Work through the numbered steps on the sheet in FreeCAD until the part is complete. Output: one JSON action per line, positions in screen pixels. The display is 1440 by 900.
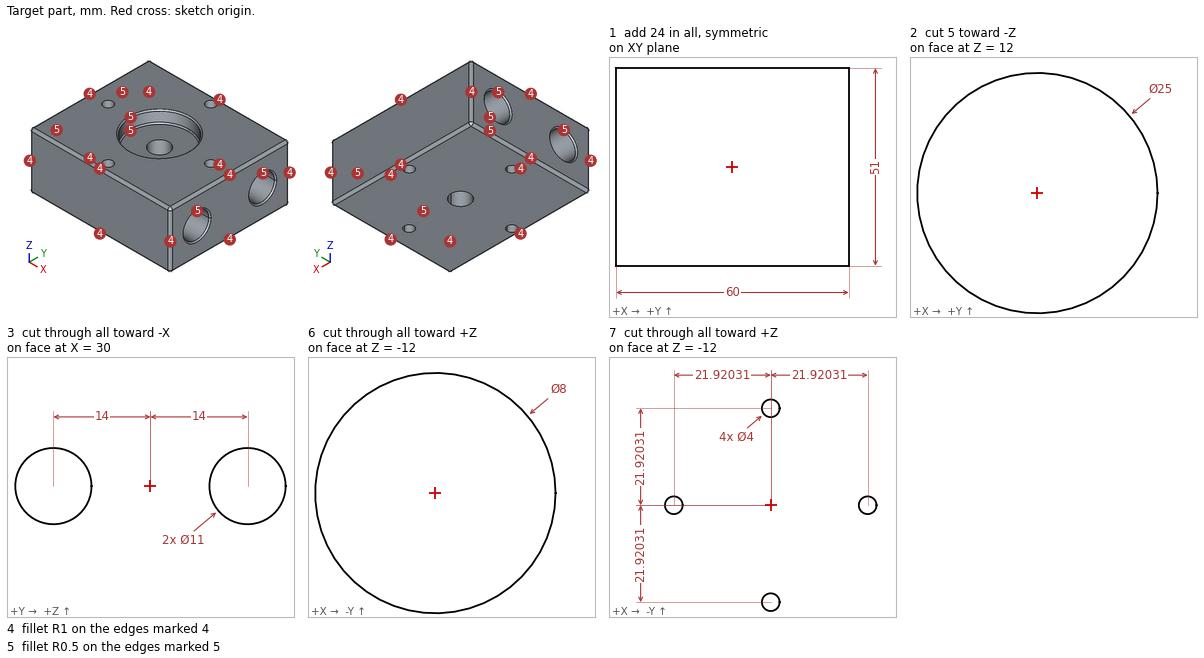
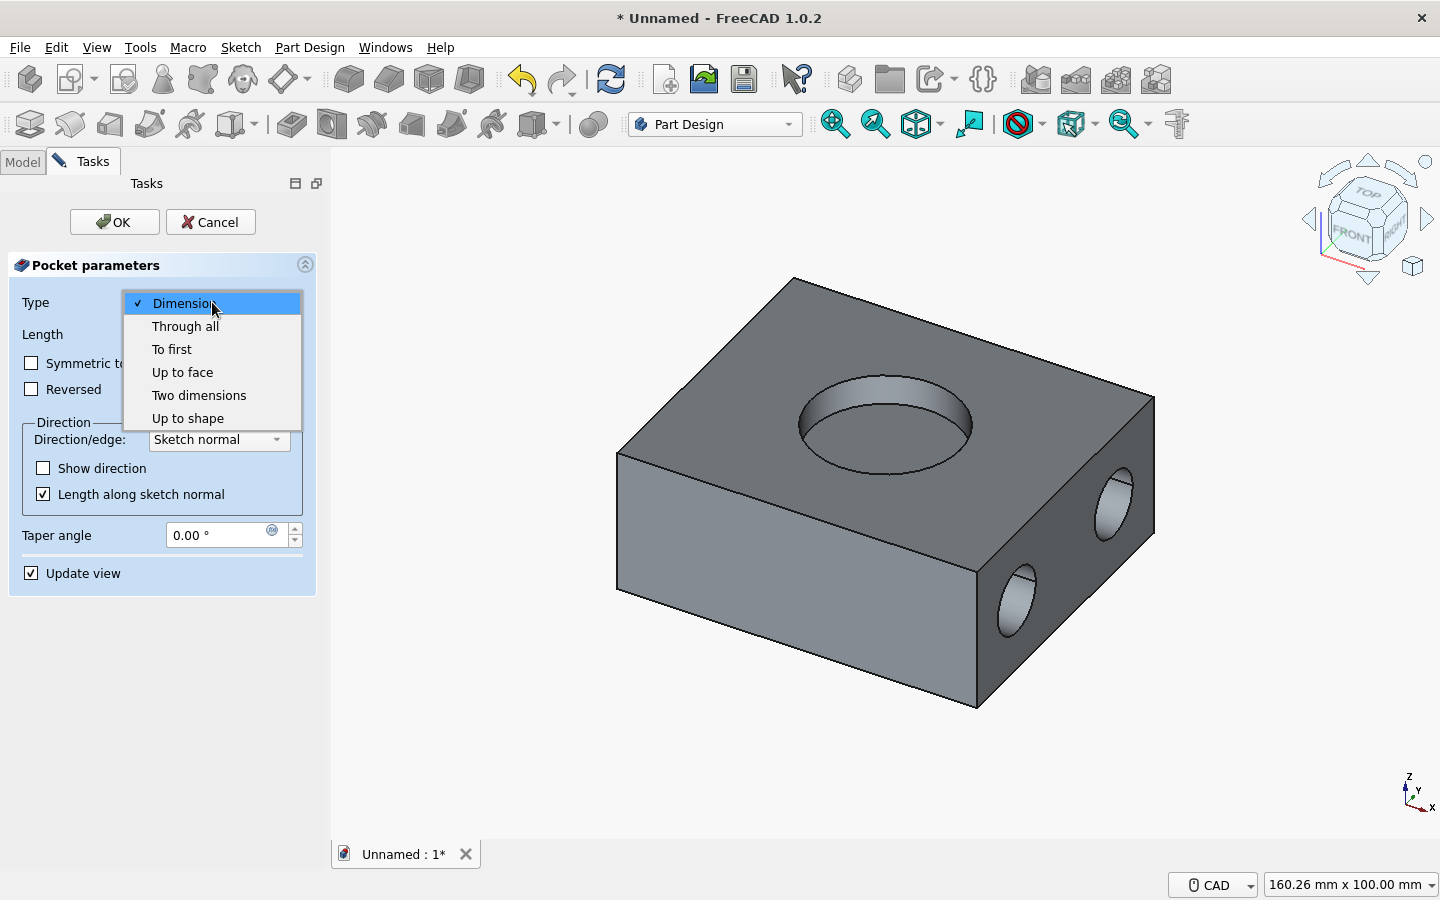
{"action": "left_click", "coordinate": [212, 326]}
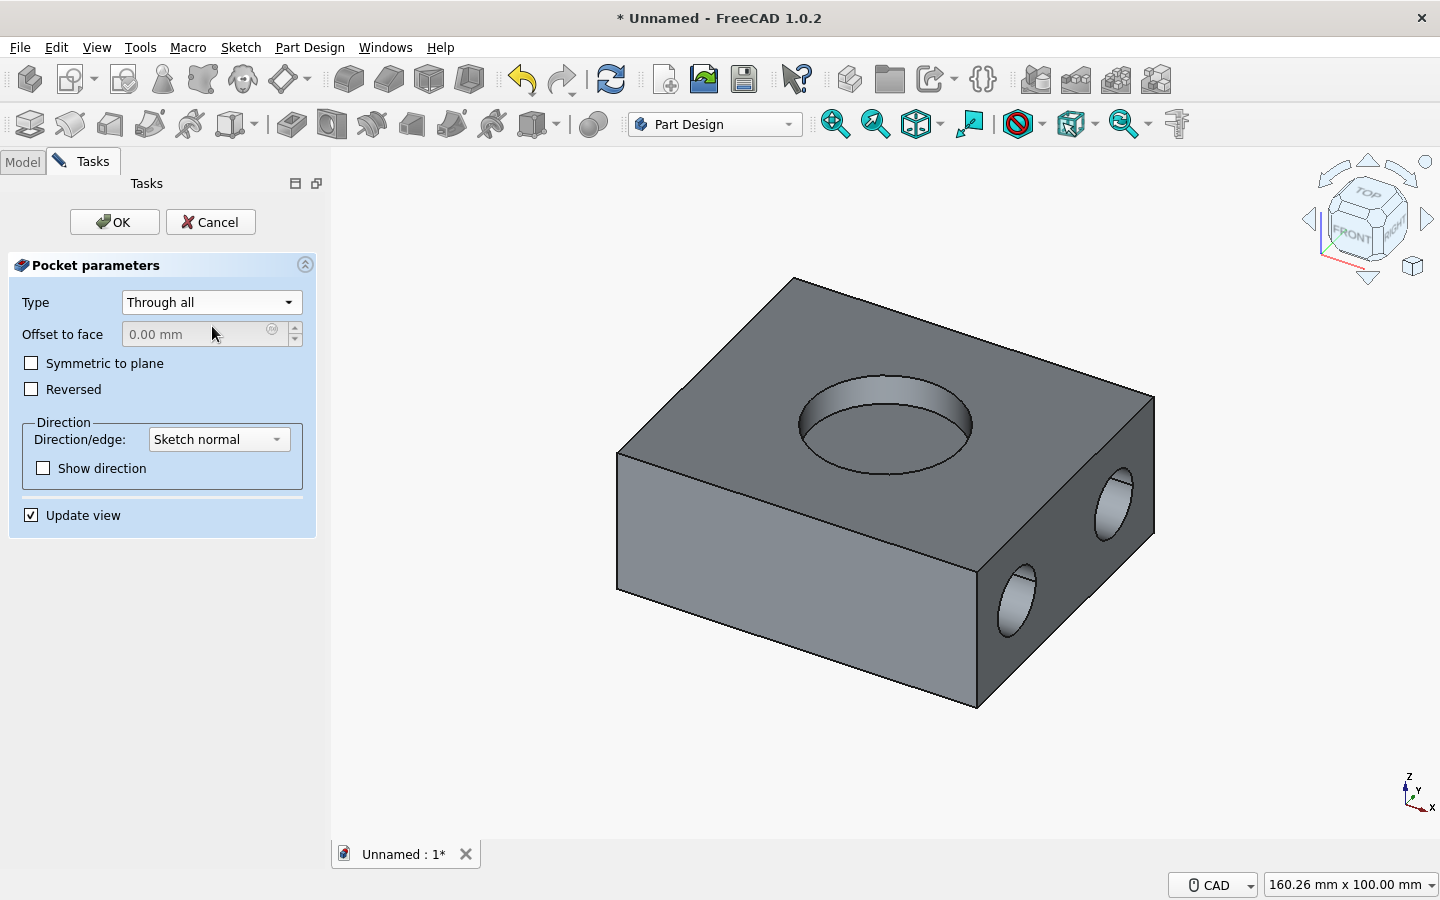
{"action": "left_click", "coordinate": [115, 222]}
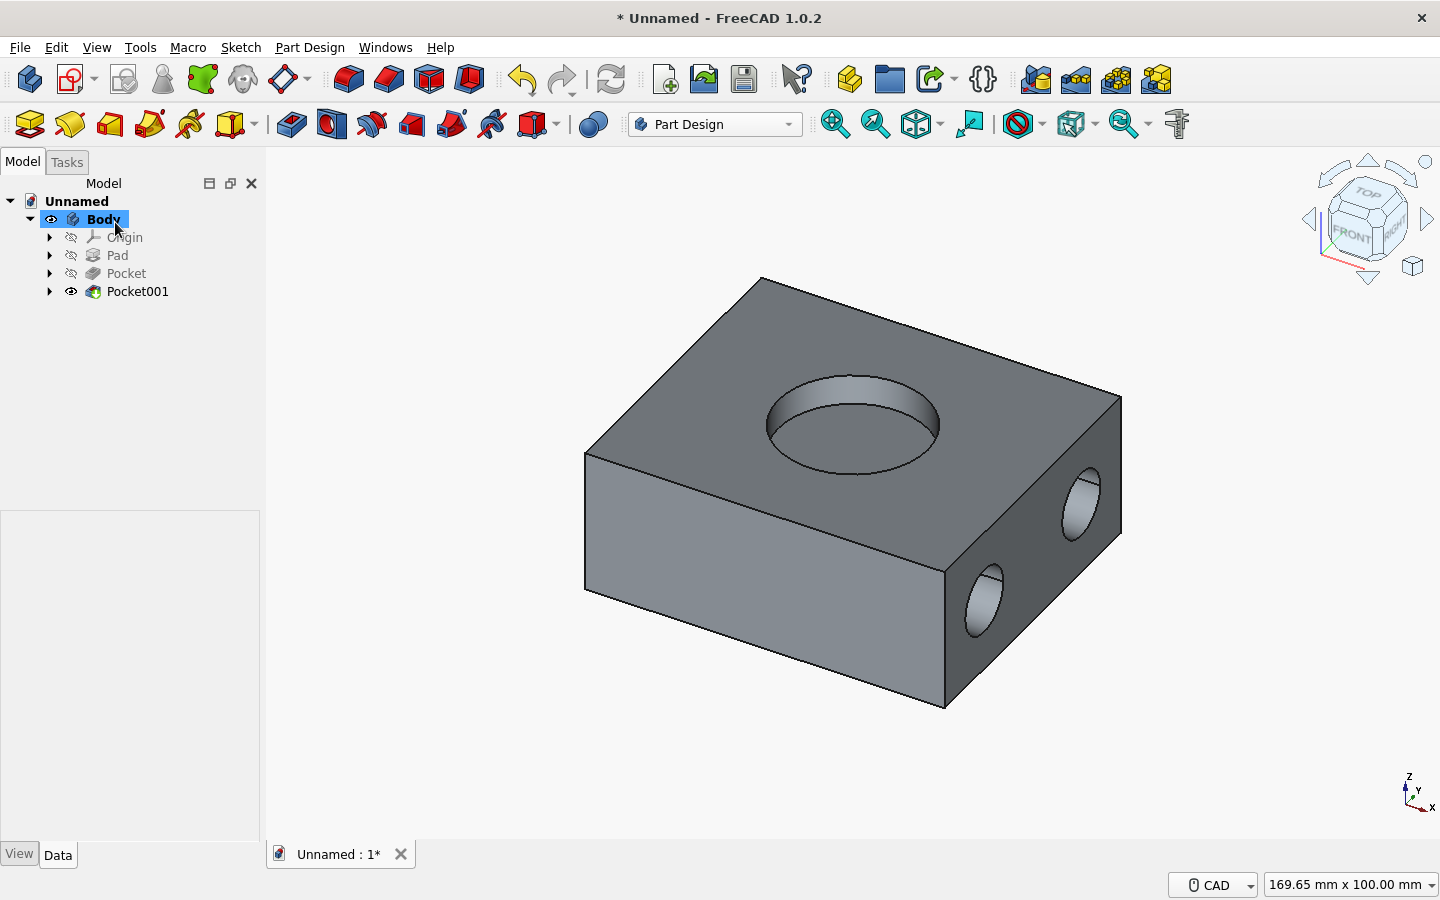
{"action": "left_click", "coordinate": [868, 614]}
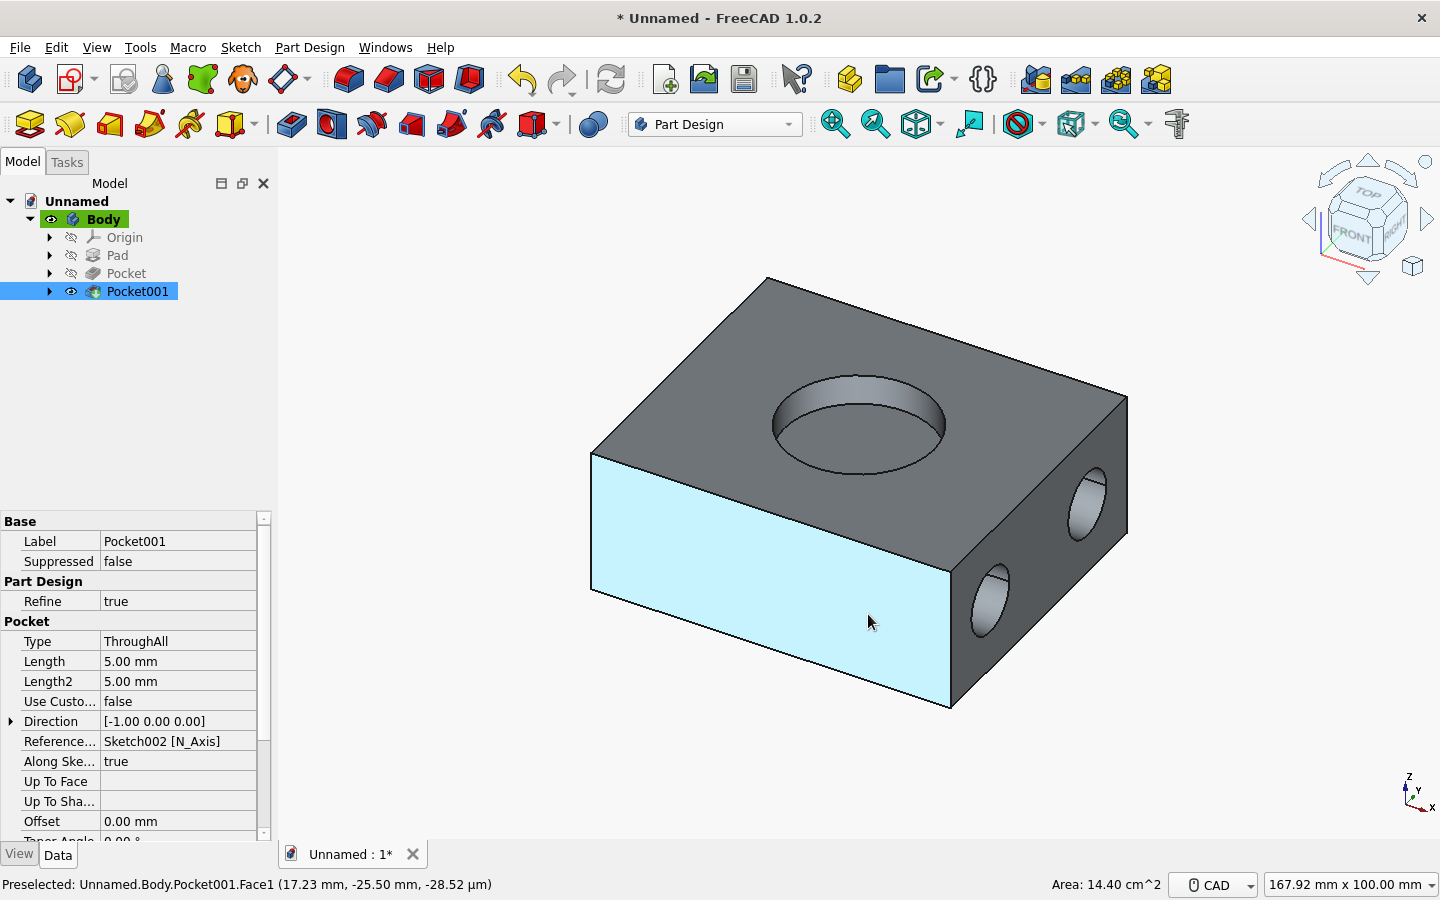
{"action": "left_click", "coordinate": [1039, 484], "text": "ctrl"}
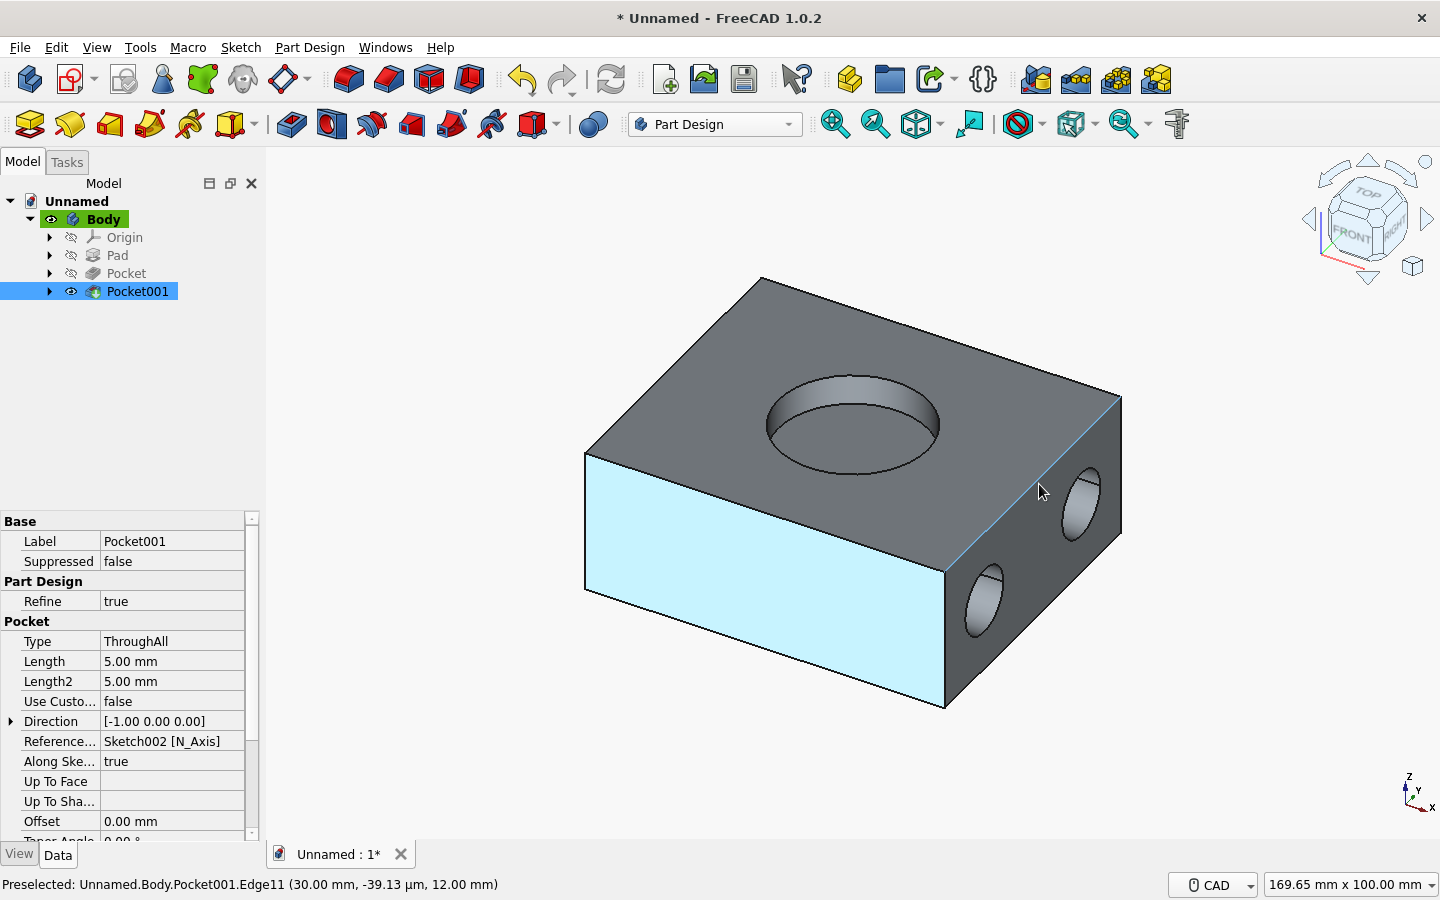
{"action": "key", "text": "0"}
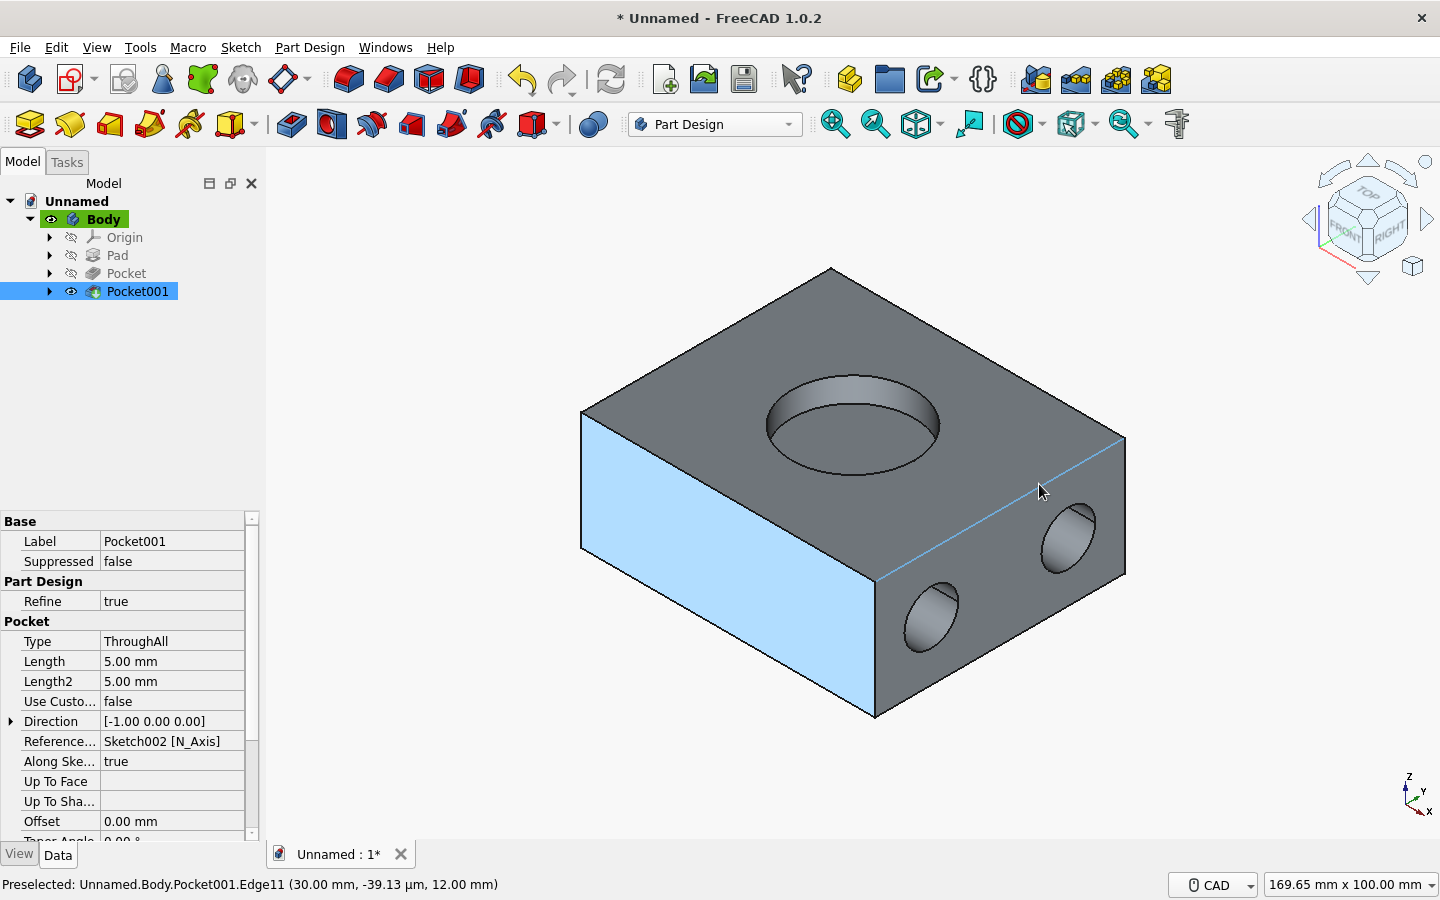
{"action": "key", "text": "2"}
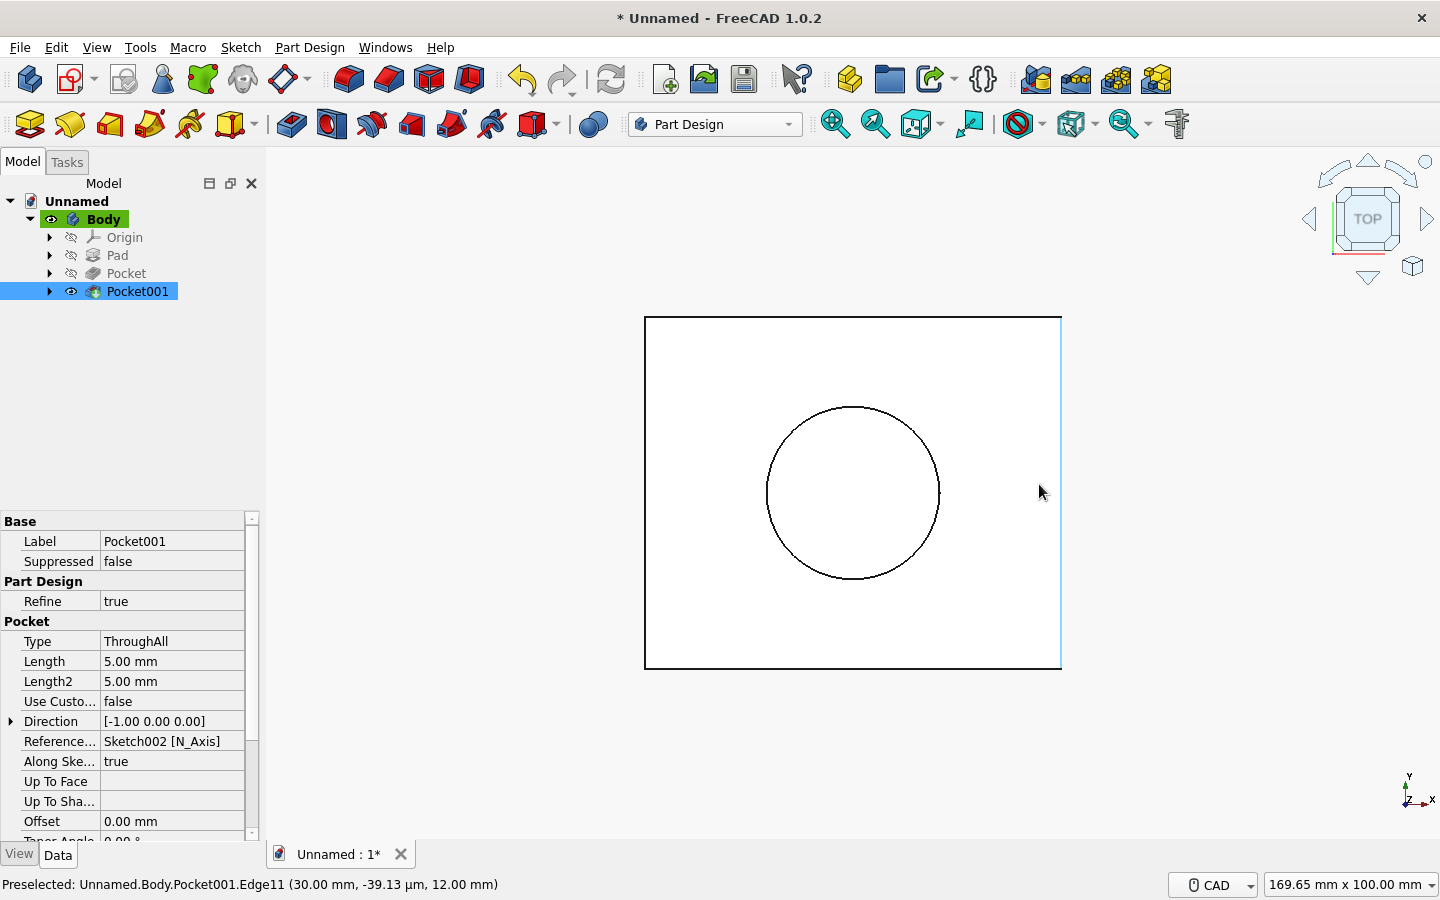
{"action": "left_click", "coordinate": [645, 492], "text": "ctrl"}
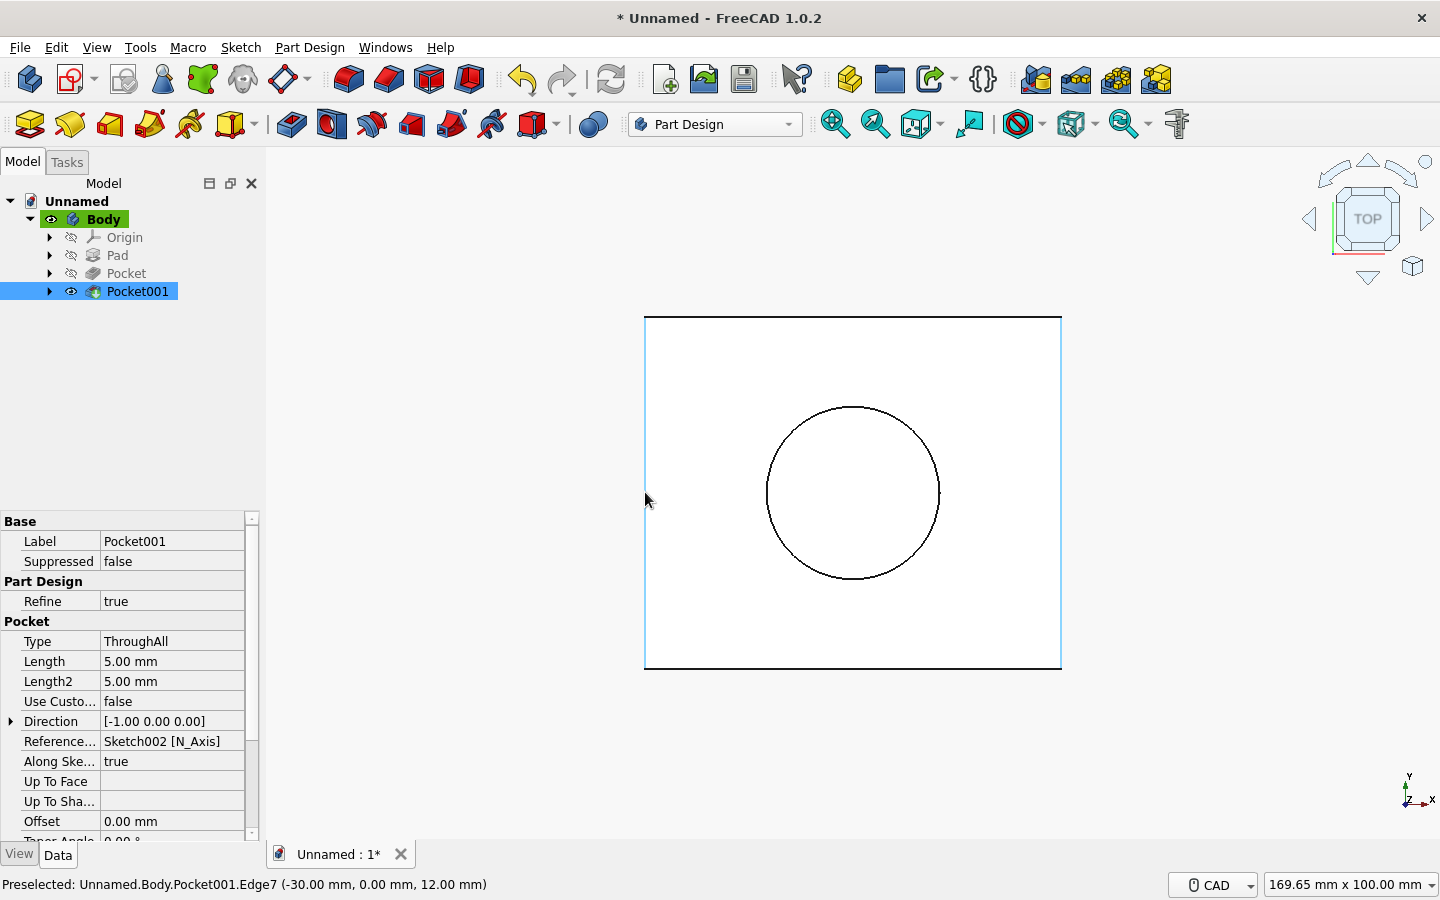
{"action": "key", "text": "1"}